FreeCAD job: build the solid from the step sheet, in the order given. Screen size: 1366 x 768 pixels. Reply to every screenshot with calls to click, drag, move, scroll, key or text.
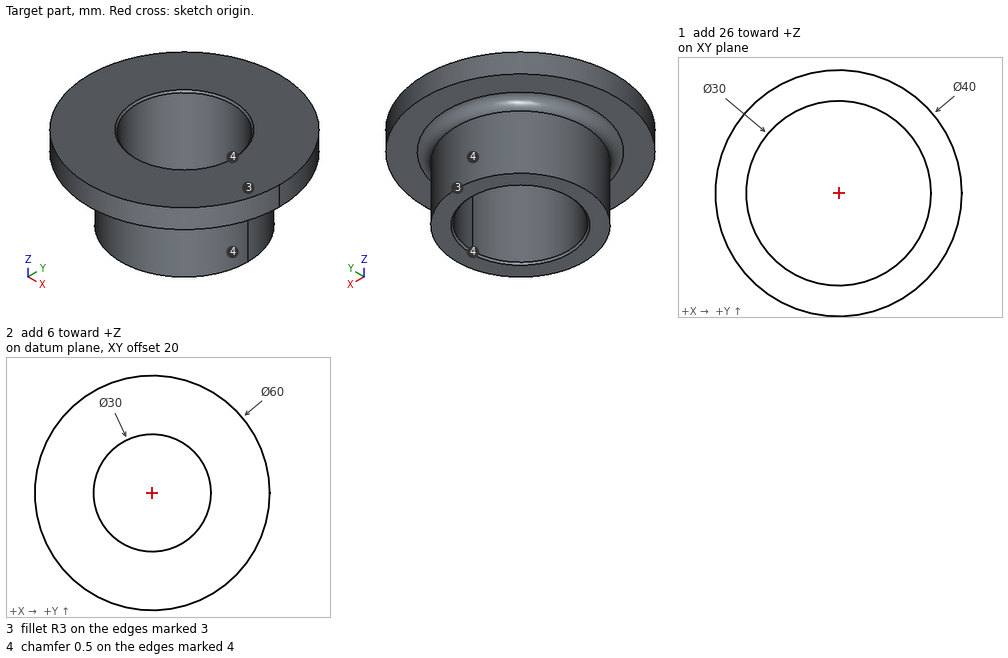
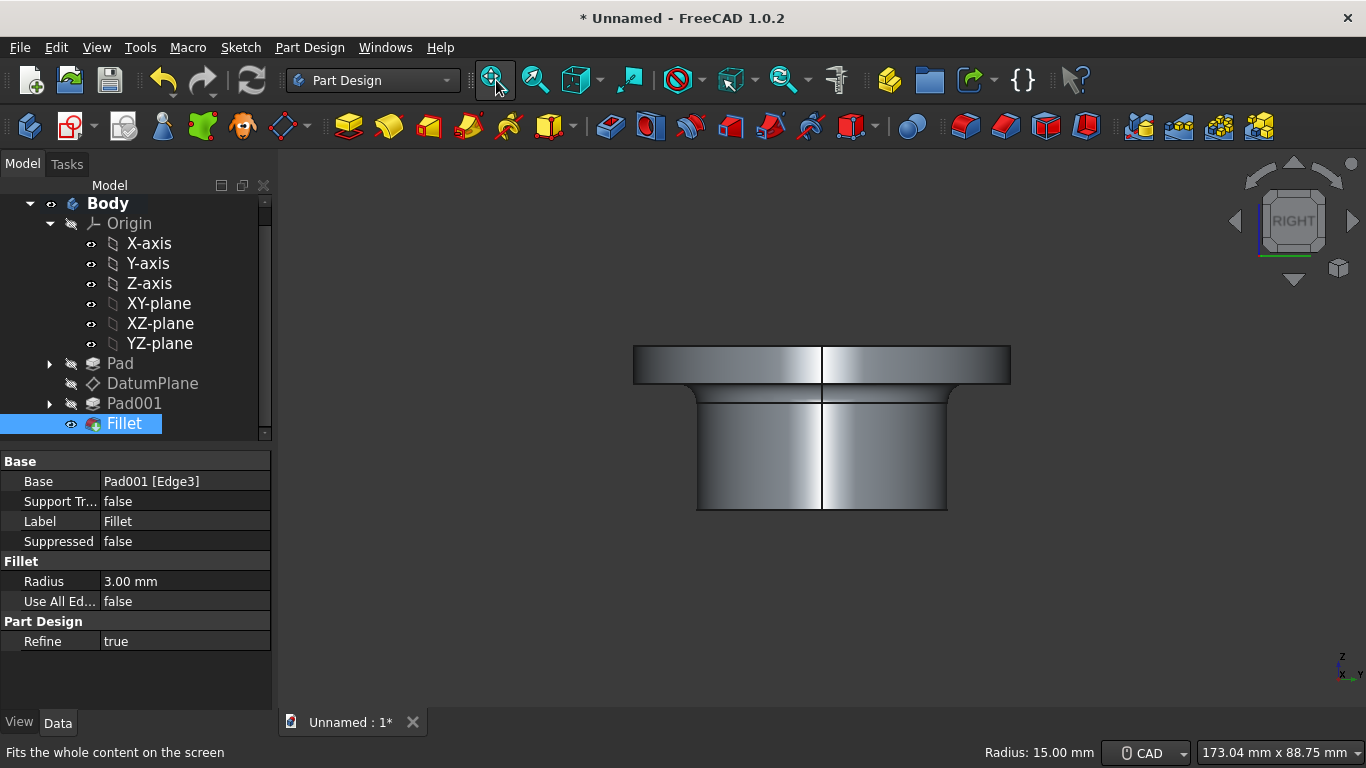
key(5)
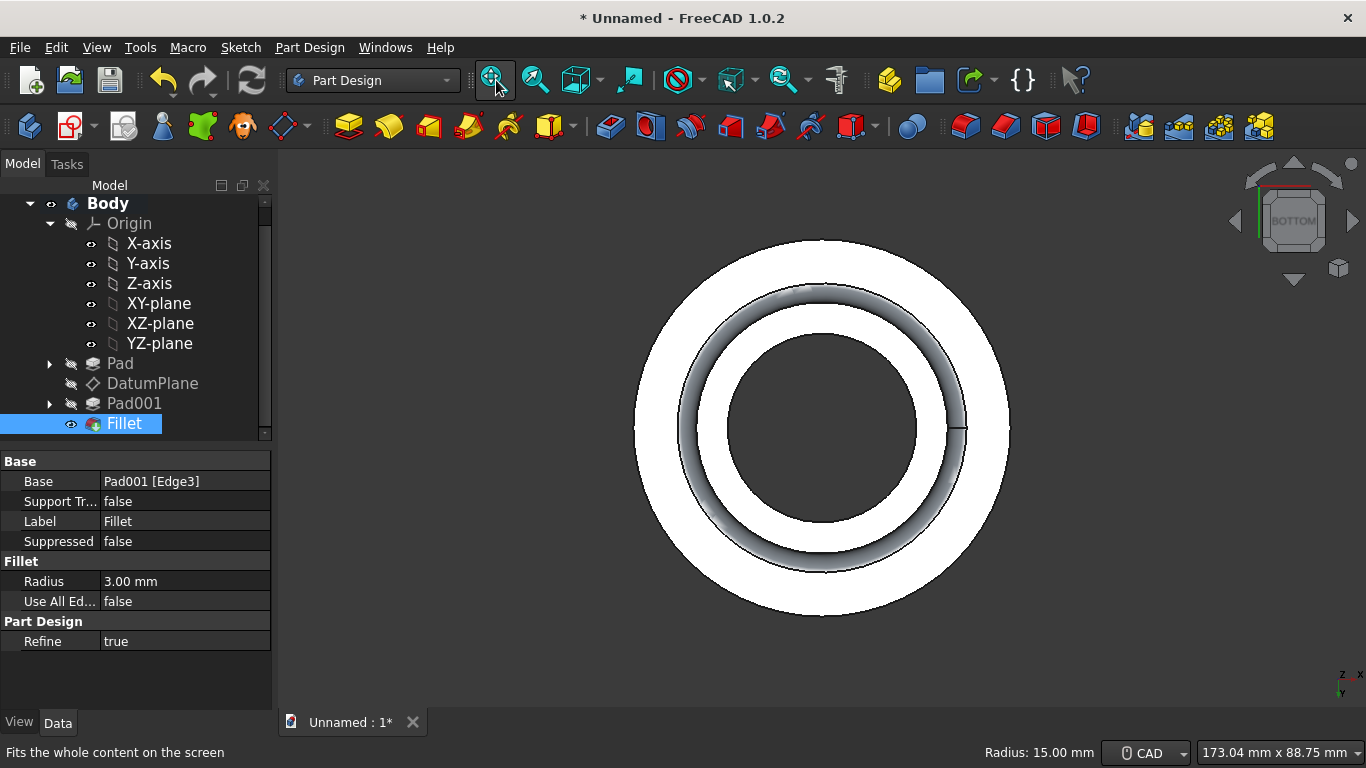
click(728, 427, ctrl)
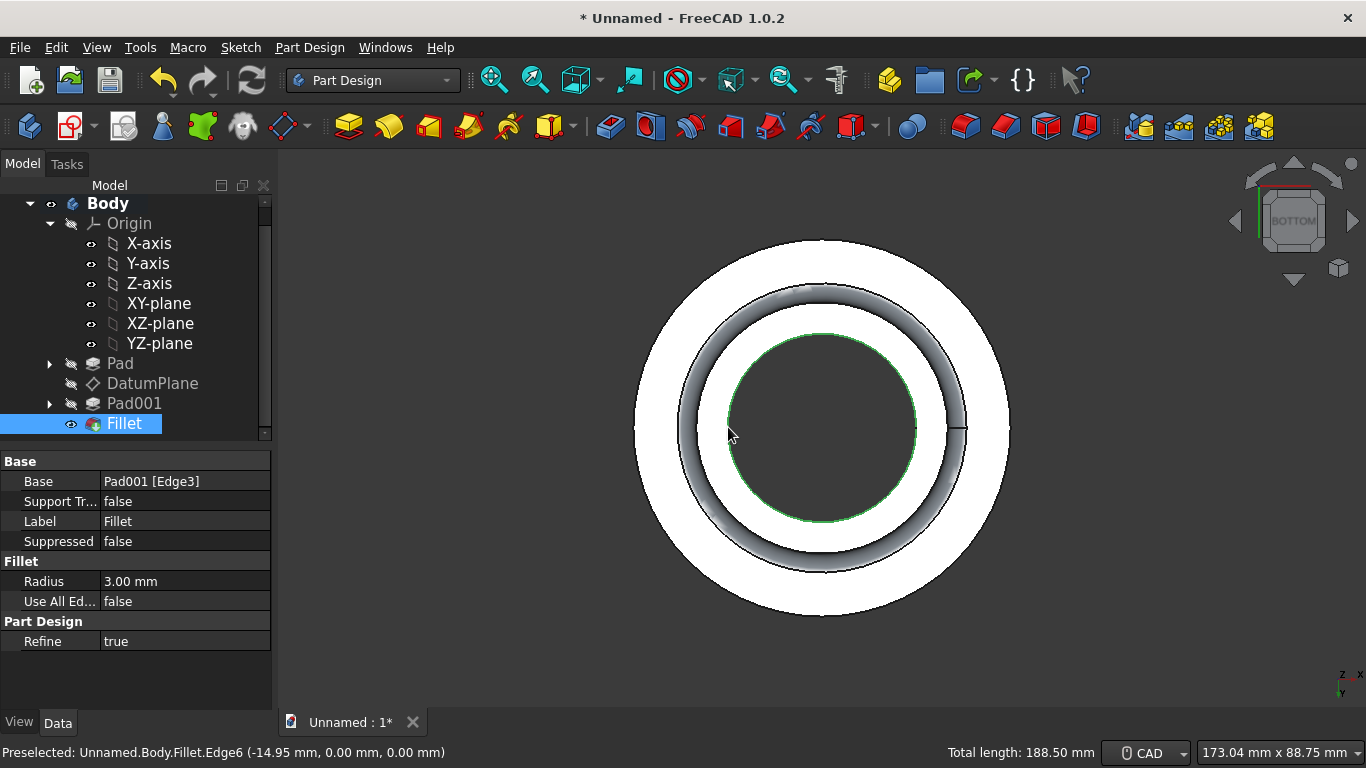
click(1006, 126)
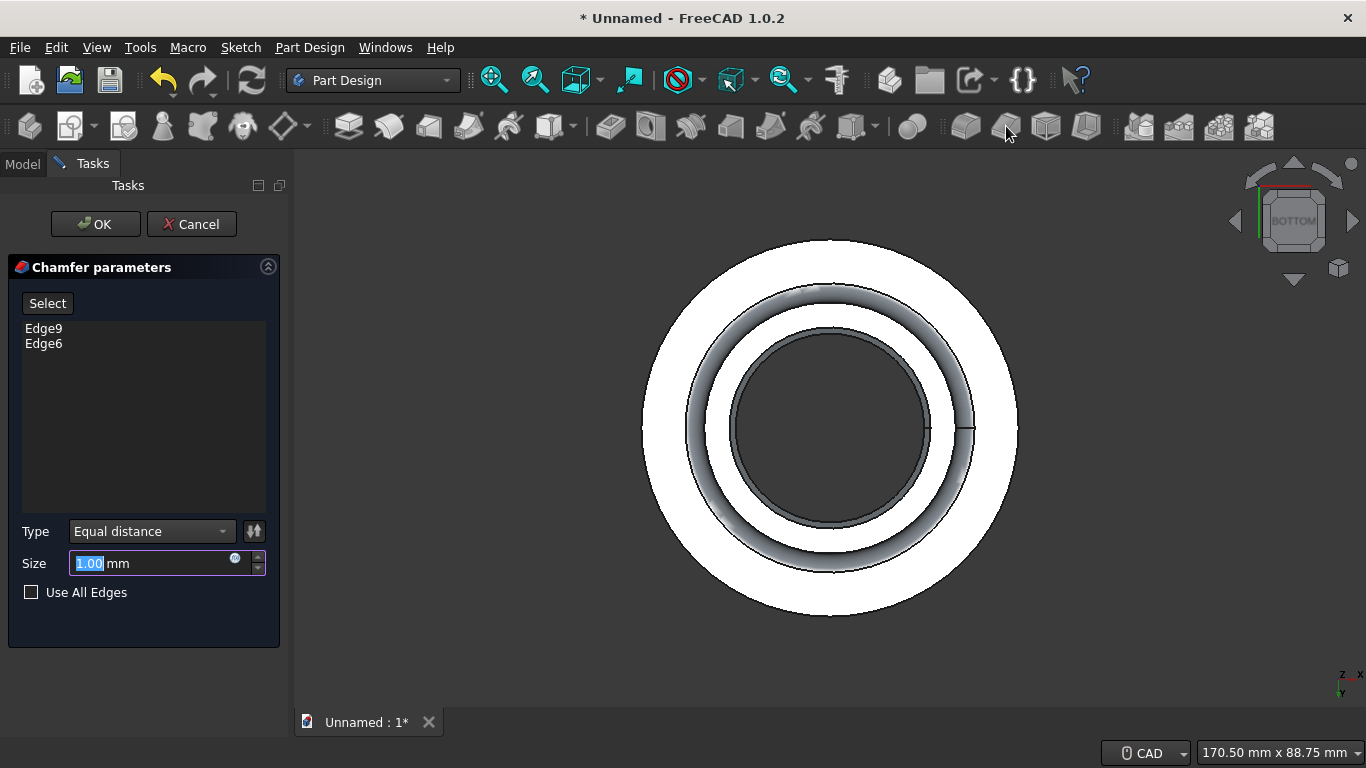
text(0.5)
key(Tab)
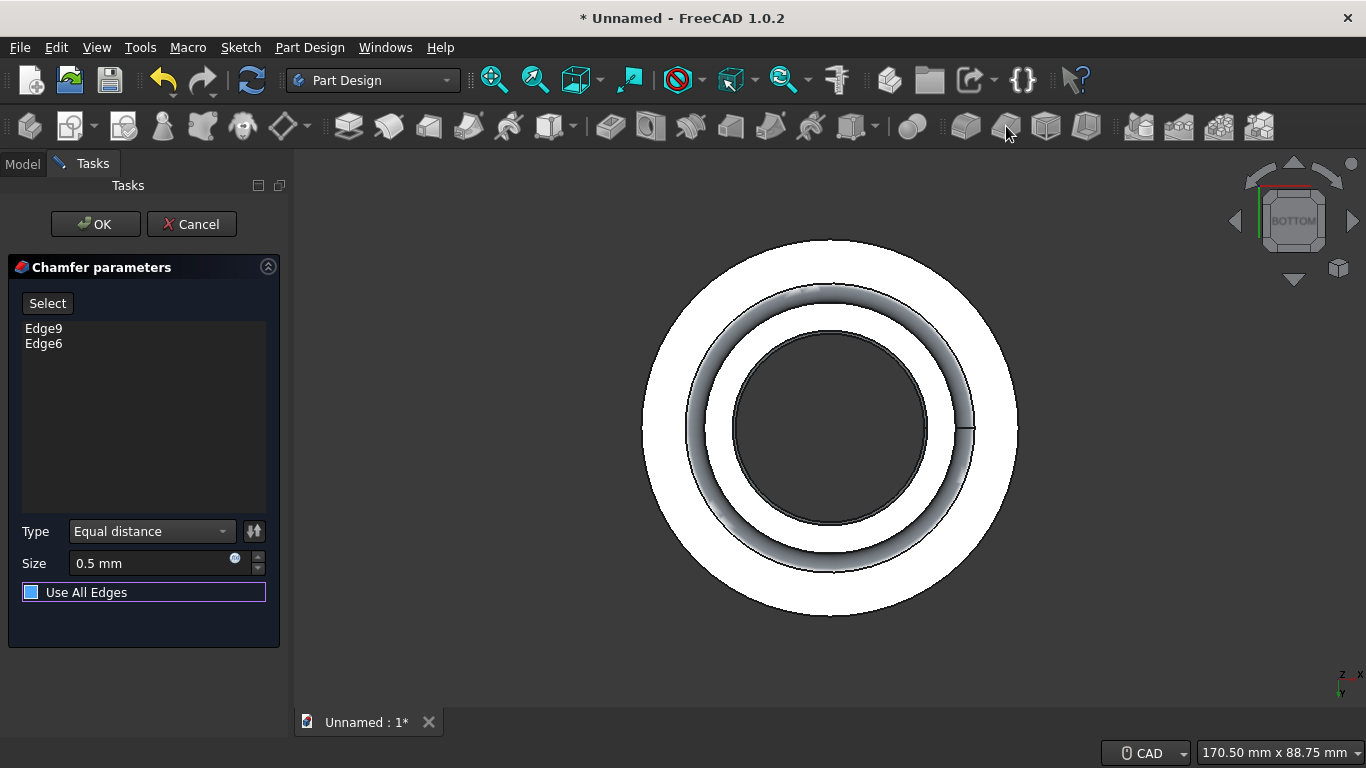
click(96, 224)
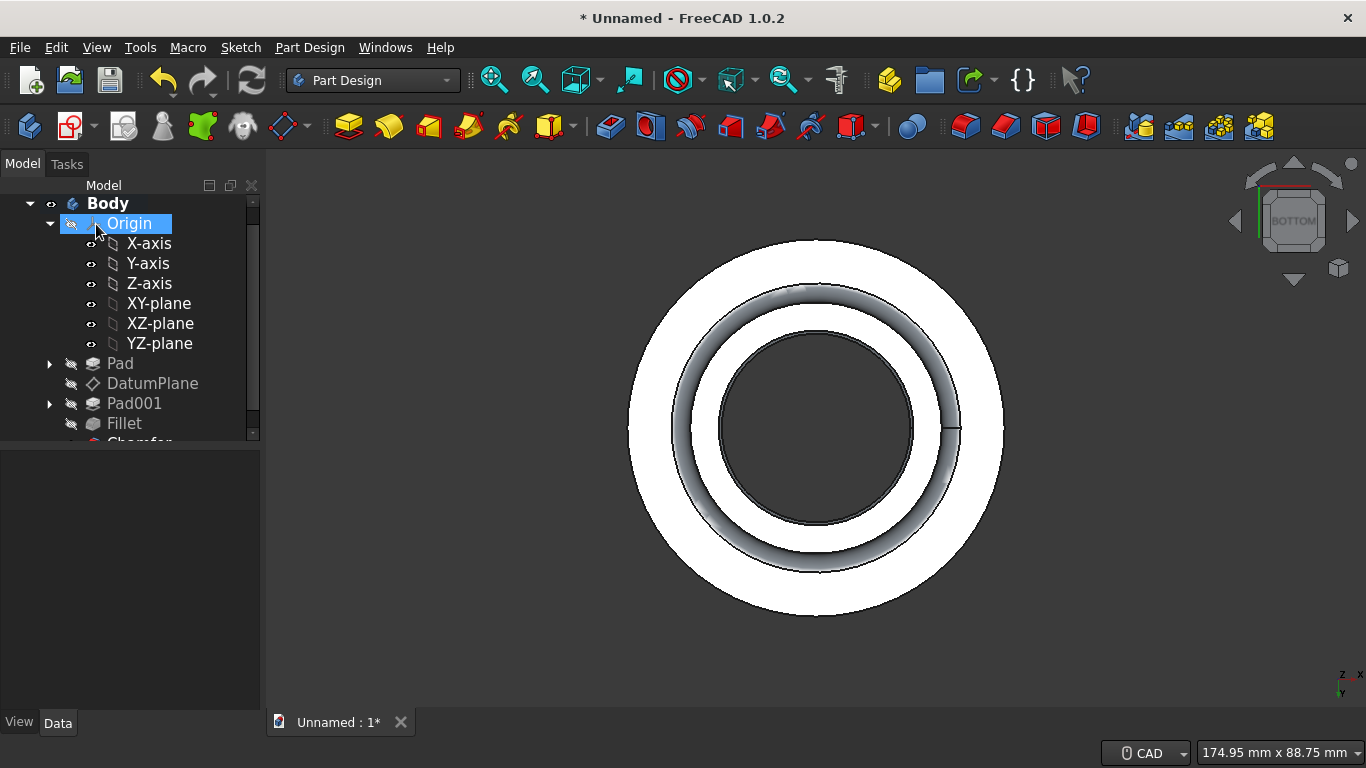
key(0)